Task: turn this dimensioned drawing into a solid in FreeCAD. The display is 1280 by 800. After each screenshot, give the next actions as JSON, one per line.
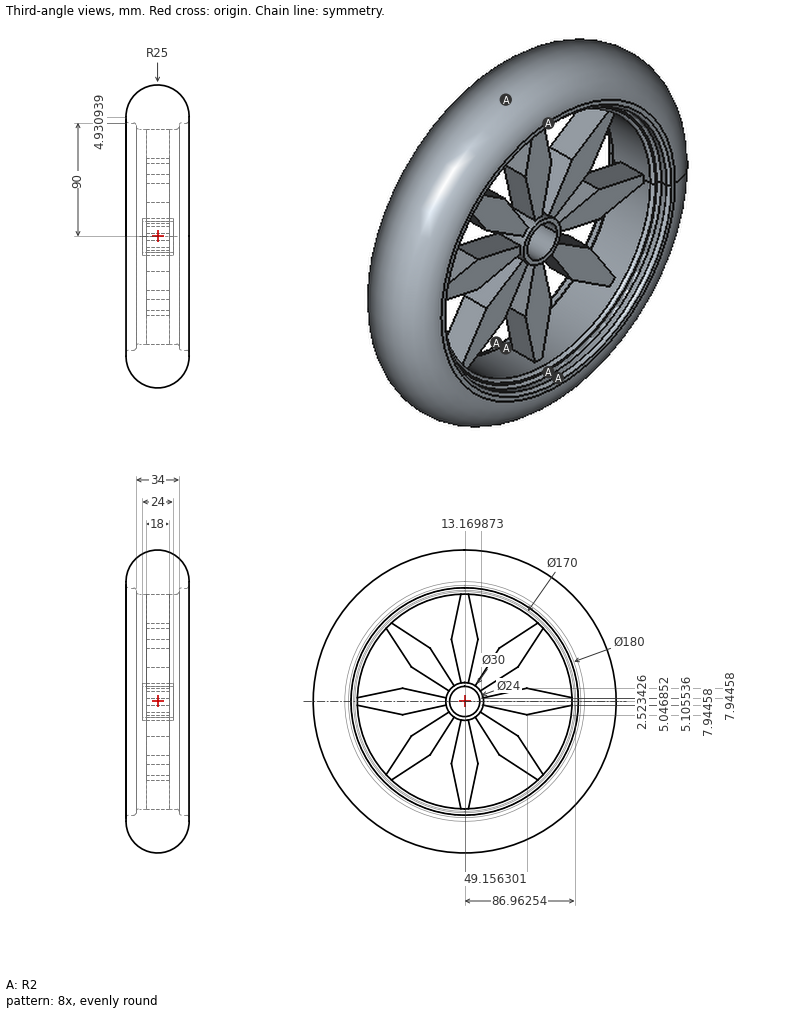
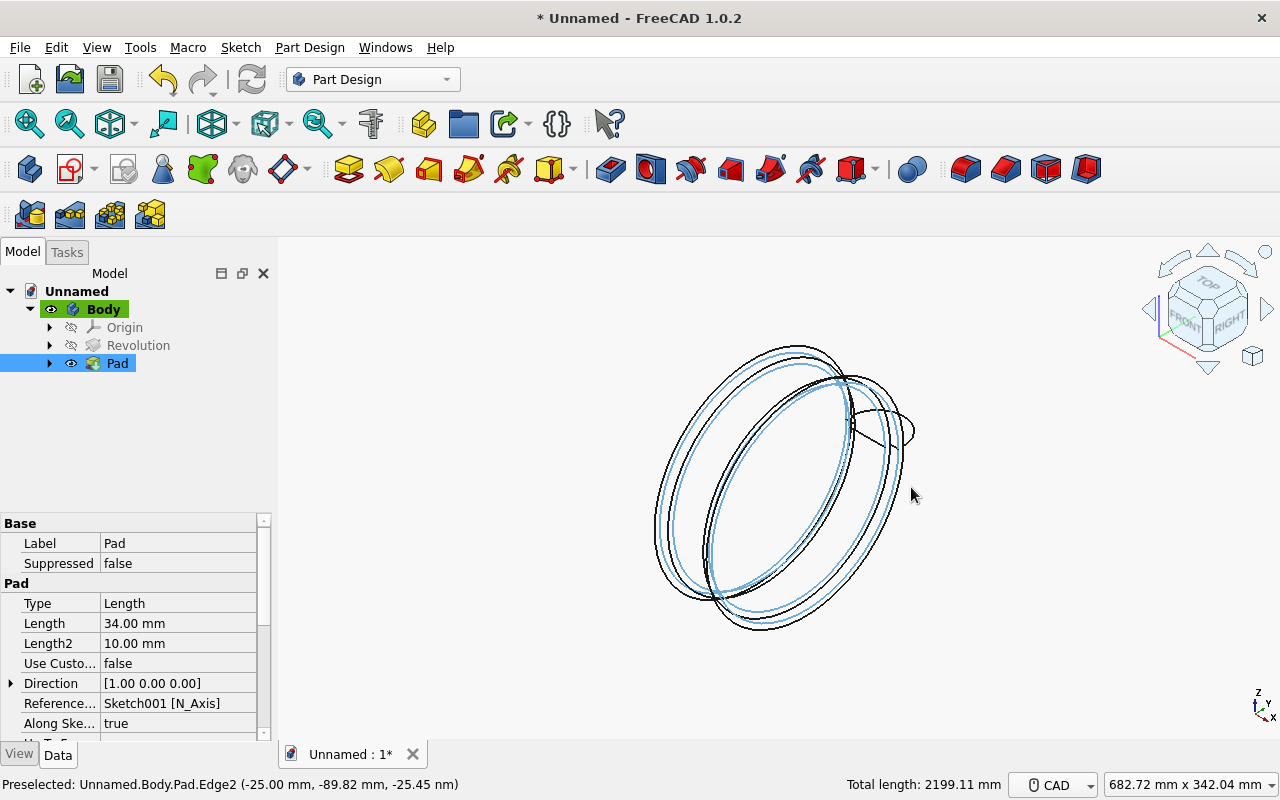
{"action": "left_click", "coordinate": [668, 531], "text": "ctrl"}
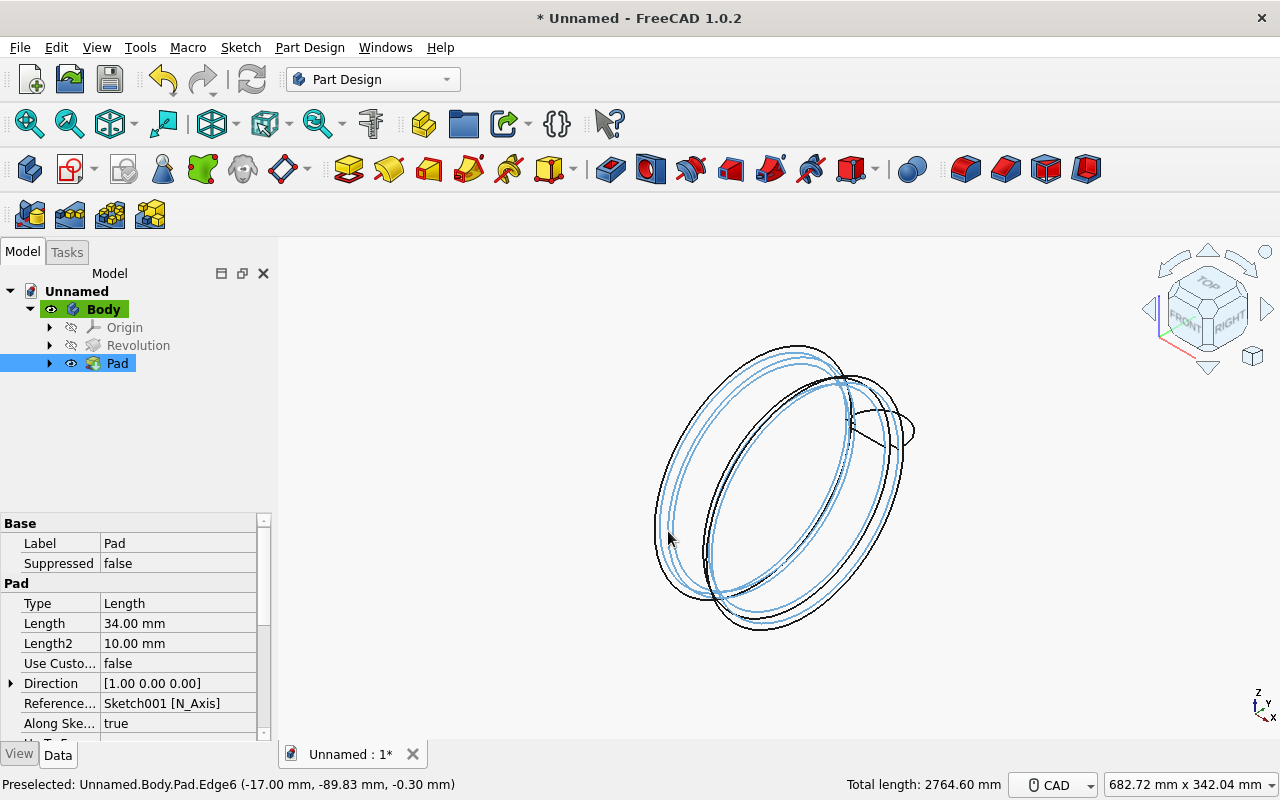
{"action": "scroll", "coordinate": [703, 551], "scroll_direction": "up", "scroll_amount": 6}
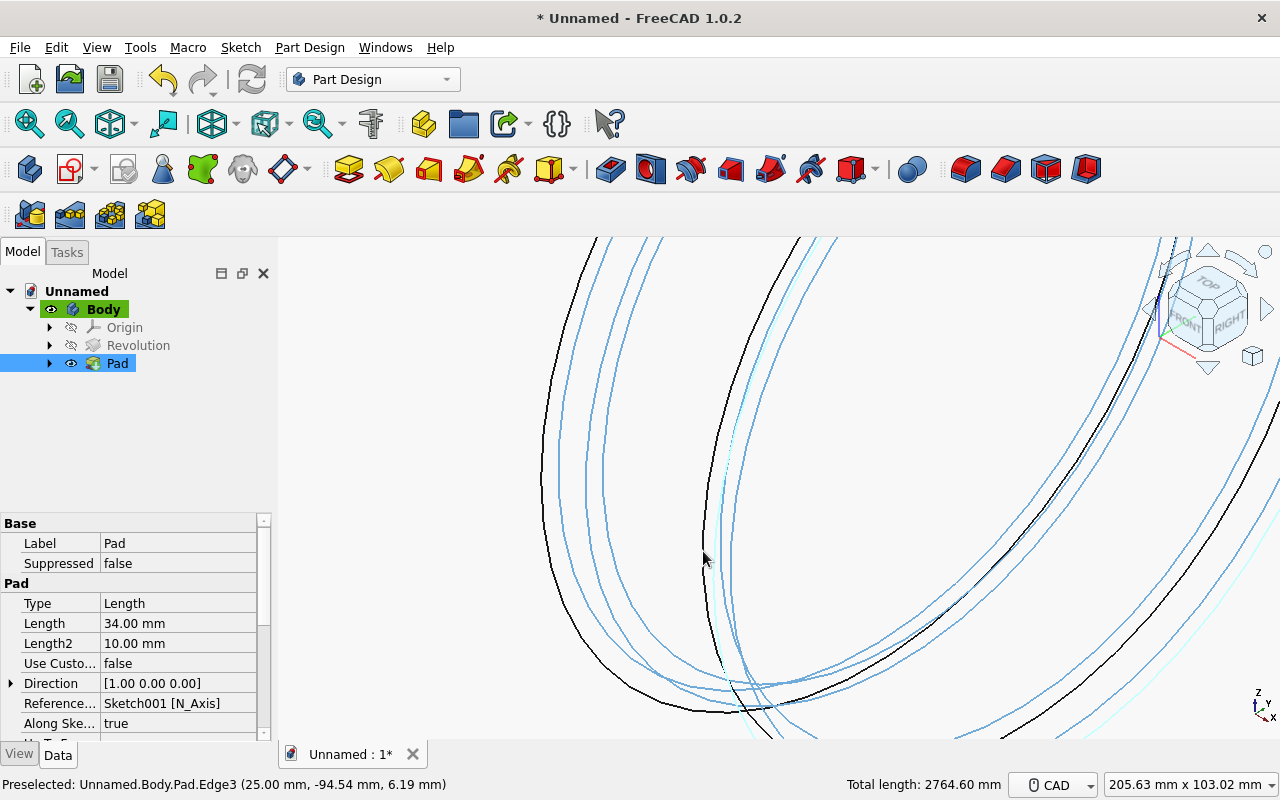
{"action": "left_click", "coordinate": [703, 552], "text": "ctrl"}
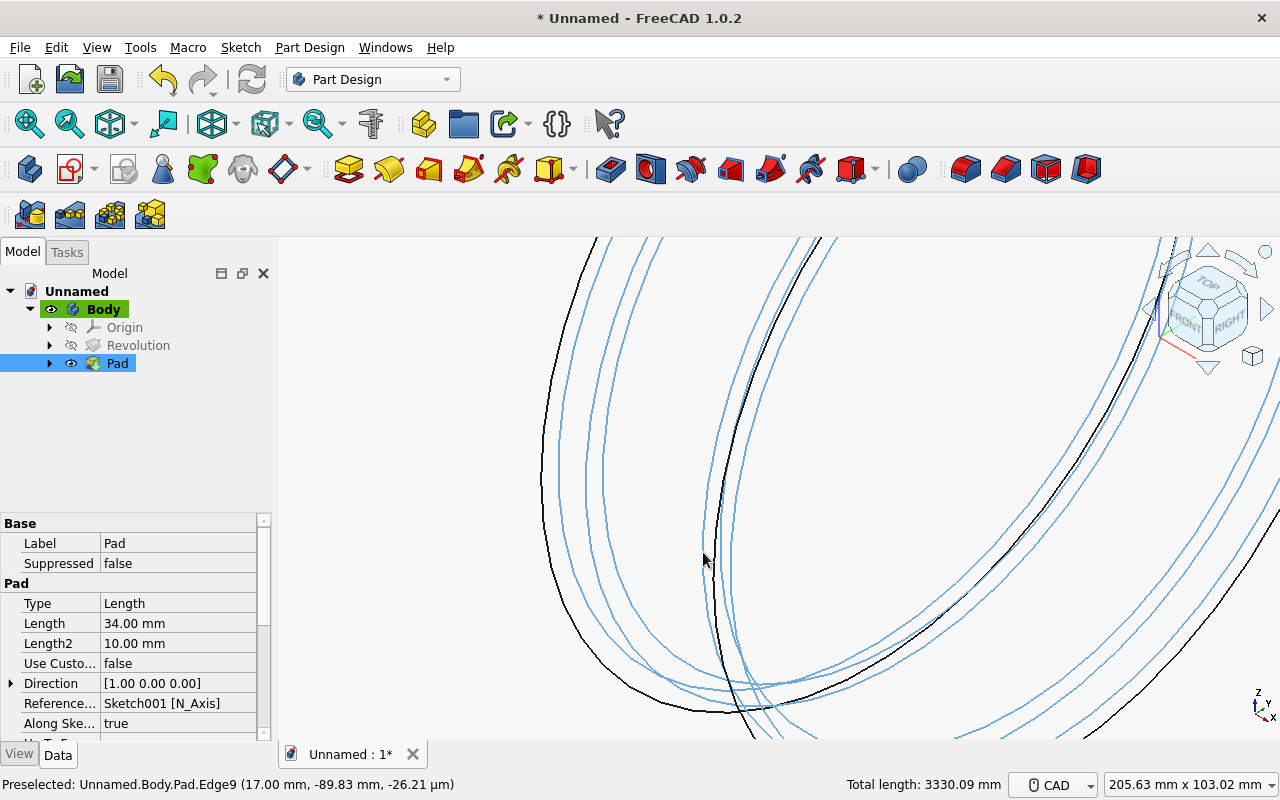
{"action": "key", "text": "v 1"}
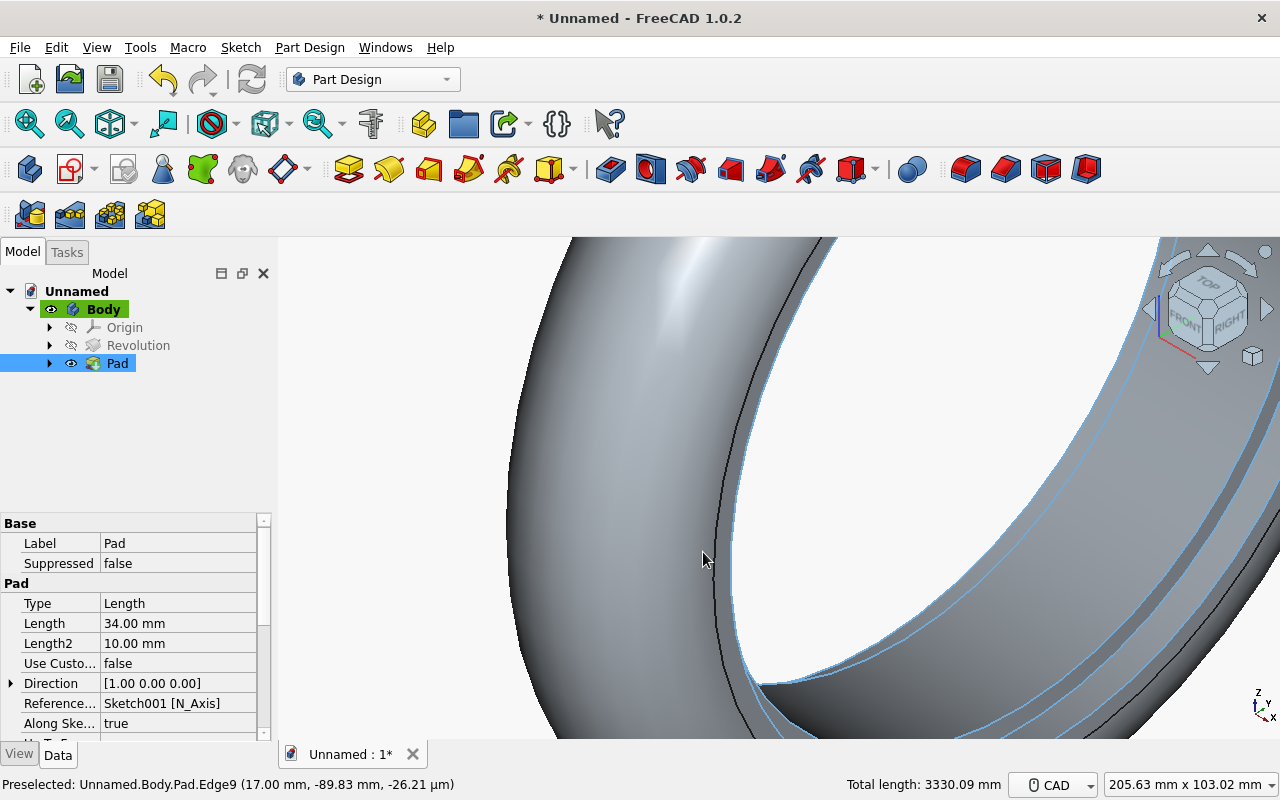
{"action": "left_click", "coordinate": [966, 170]}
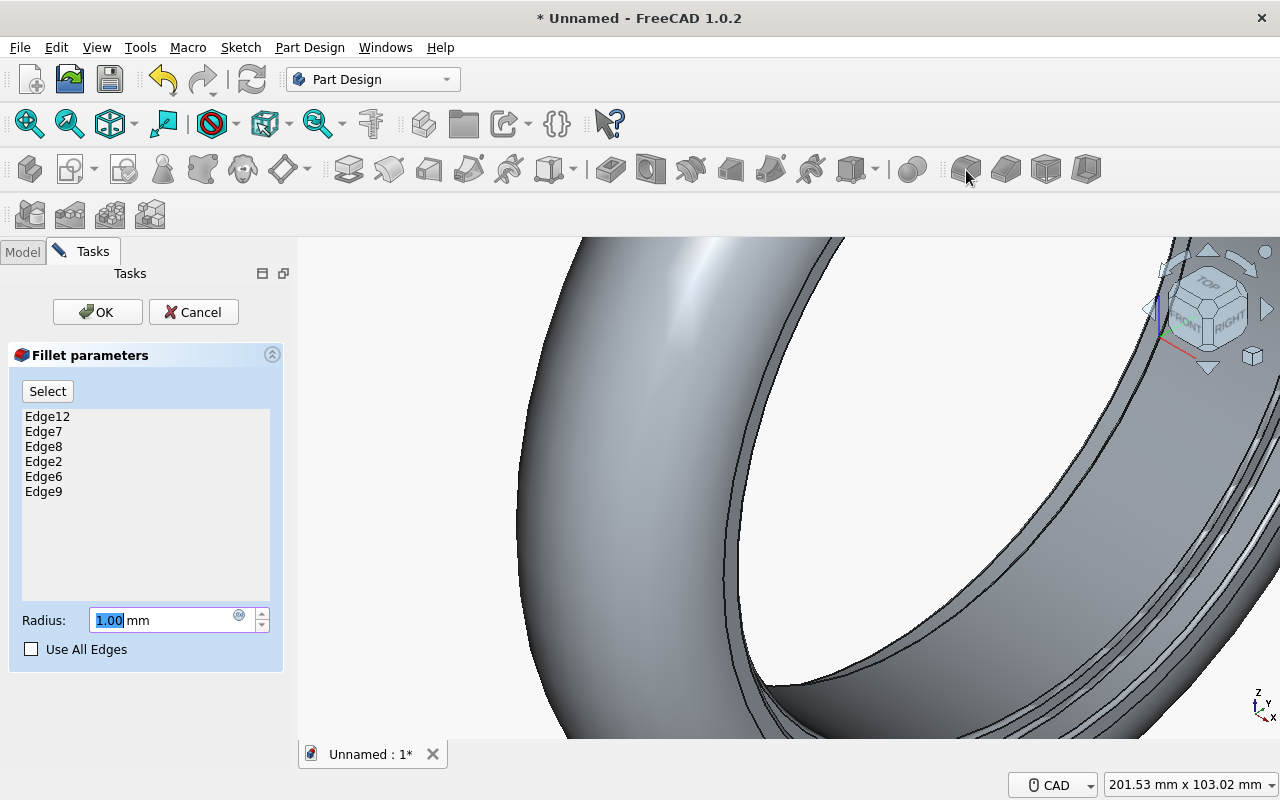
{"action": "type", "text": "2"}
{"action": "key", "text": "Tab"}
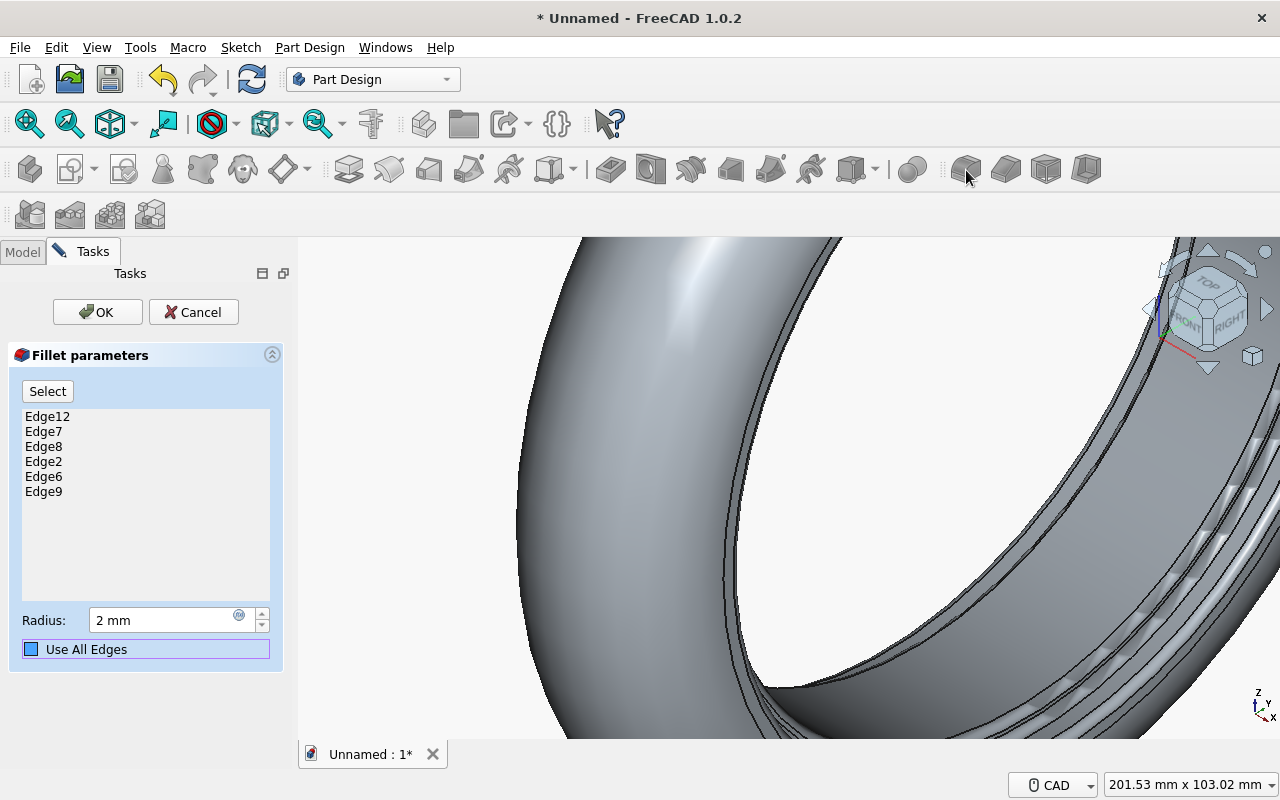
{"action": "left_click", "coordinate": [98, 312]}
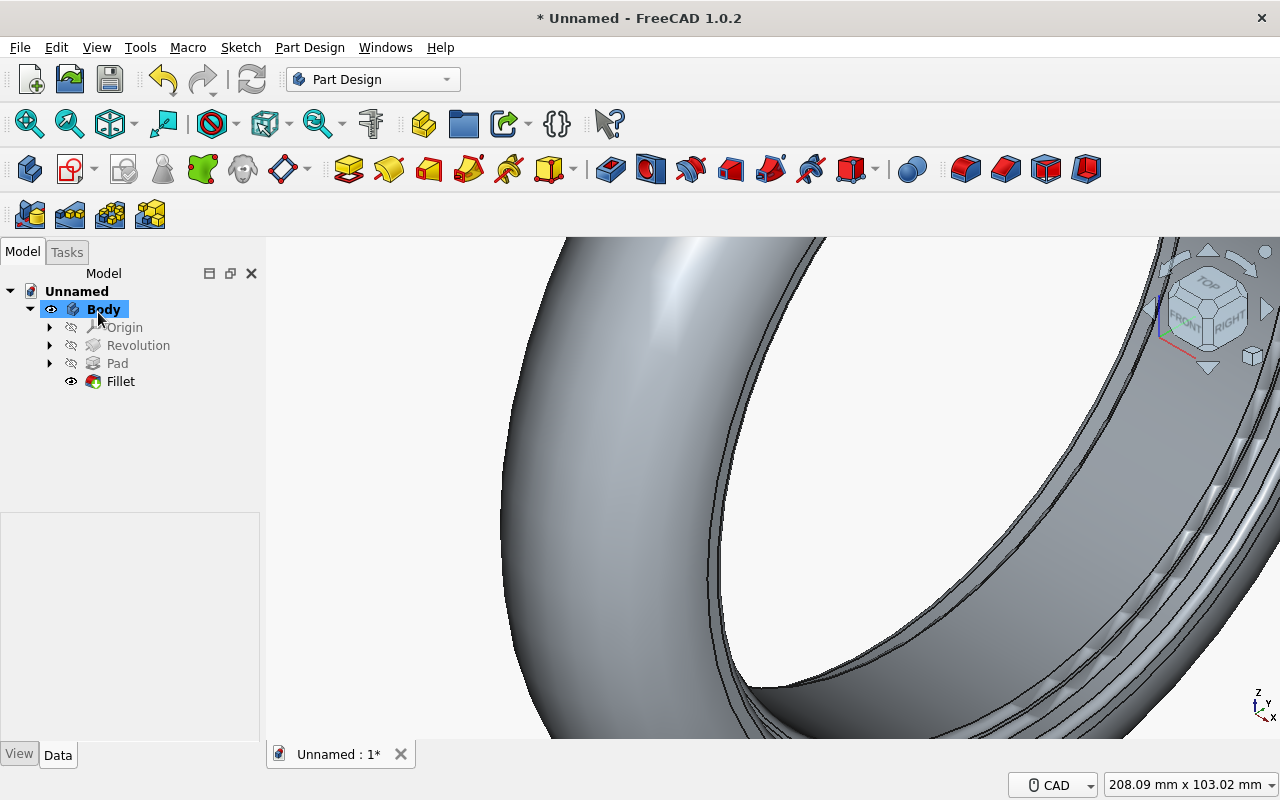
{"action": "key", "text": "v f"}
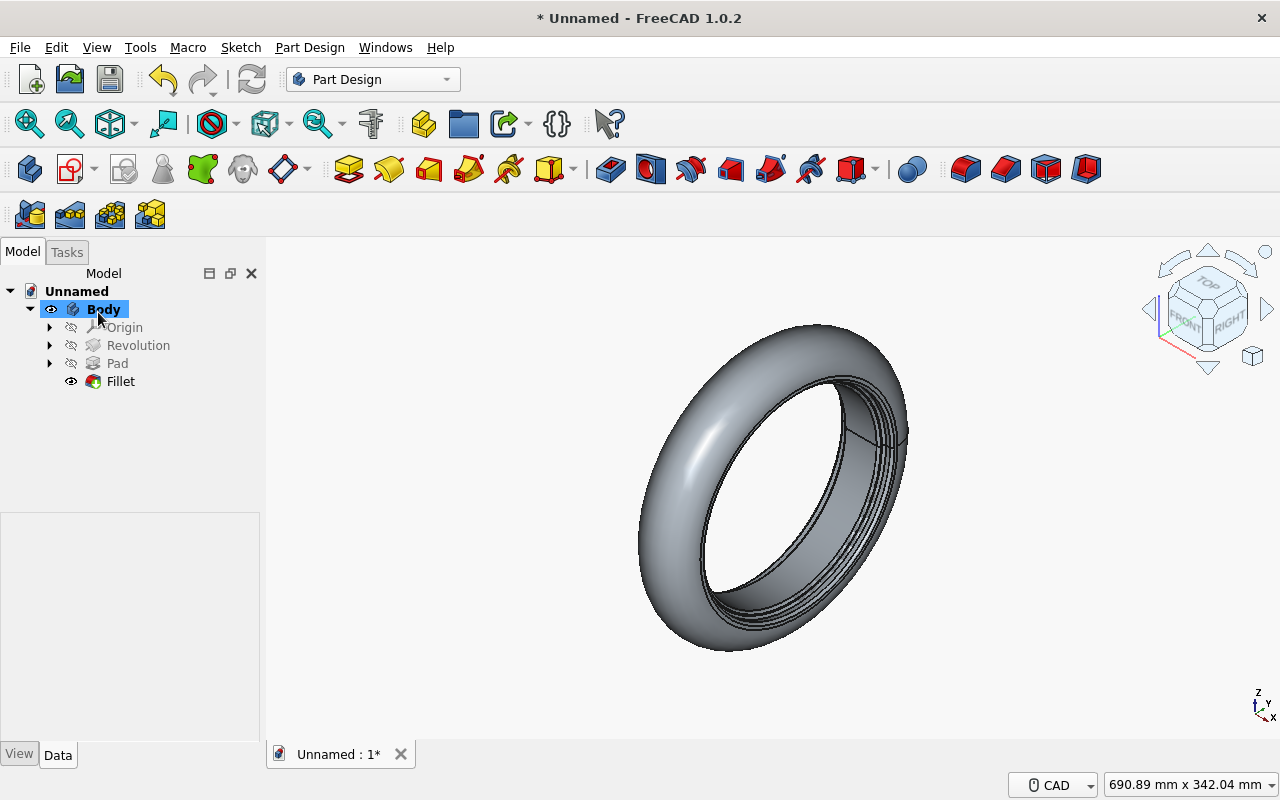
{"action": "left_click", "coordinate": [30, 170]}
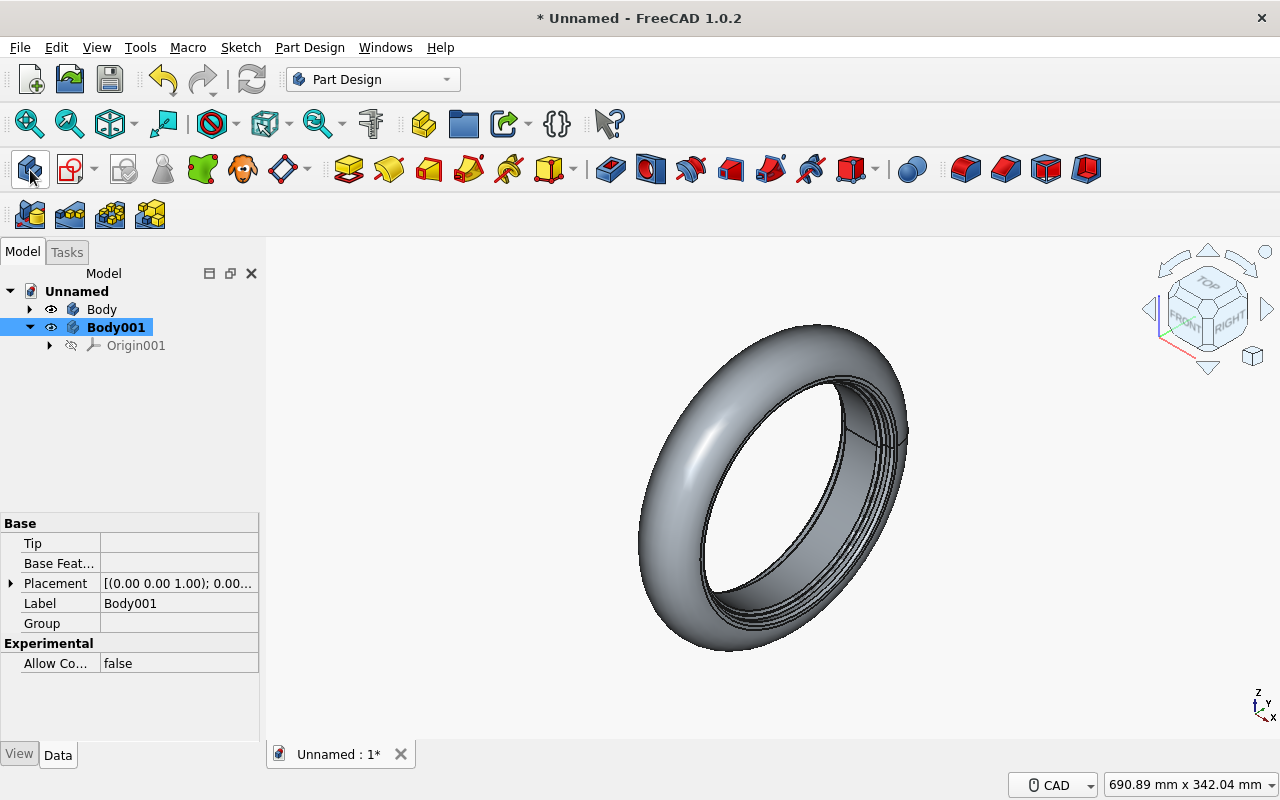
{"action": "left_click", "coordinate": [306, 699]}